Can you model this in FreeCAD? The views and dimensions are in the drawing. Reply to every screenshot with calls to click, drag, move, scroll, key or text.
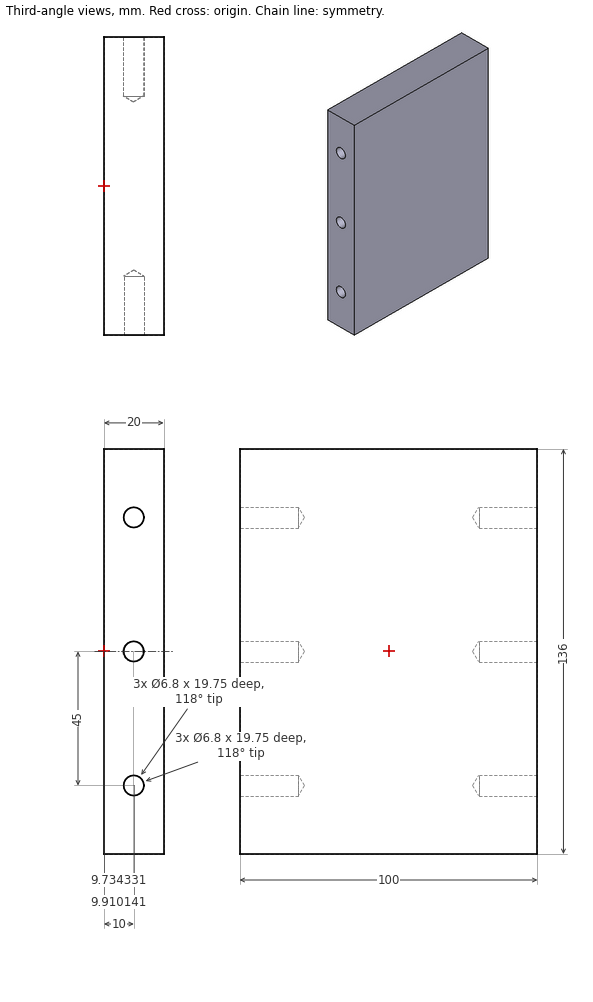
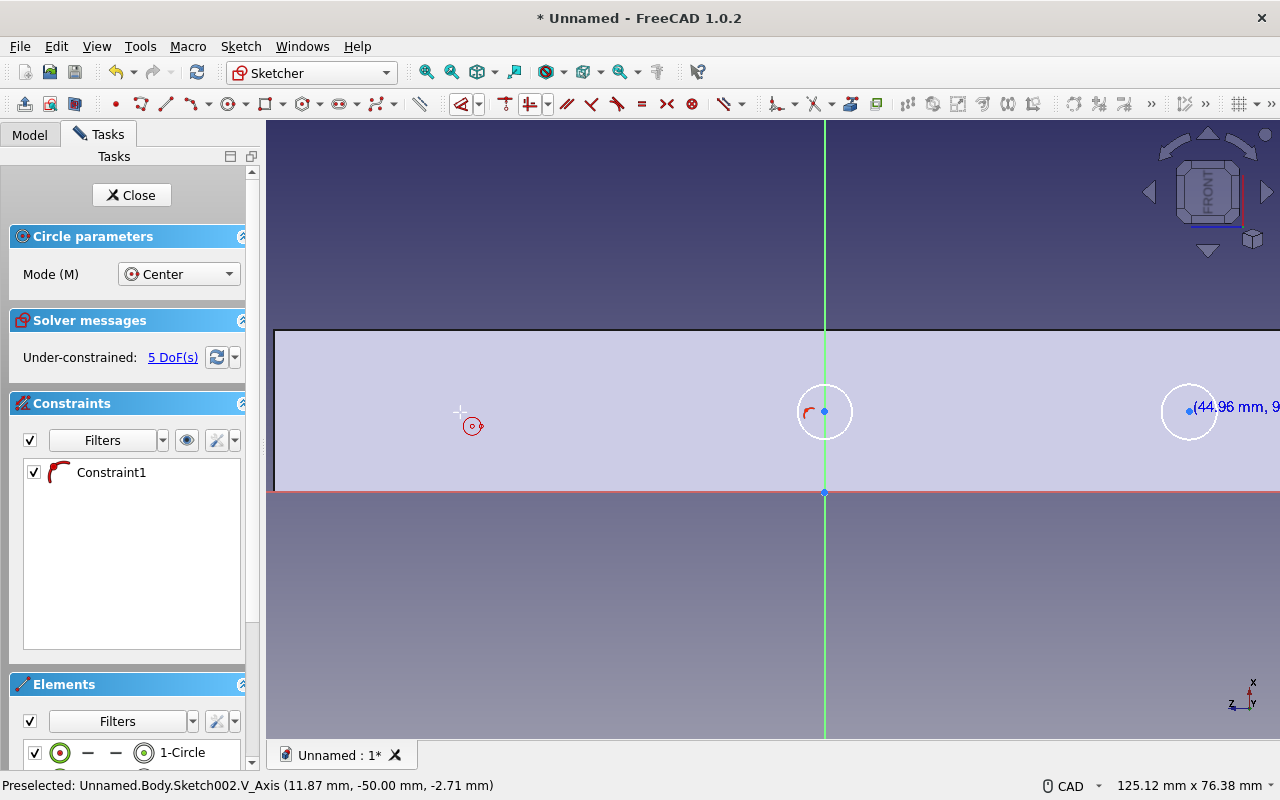
click(460, 411)
click(480, 392)
key(Escape)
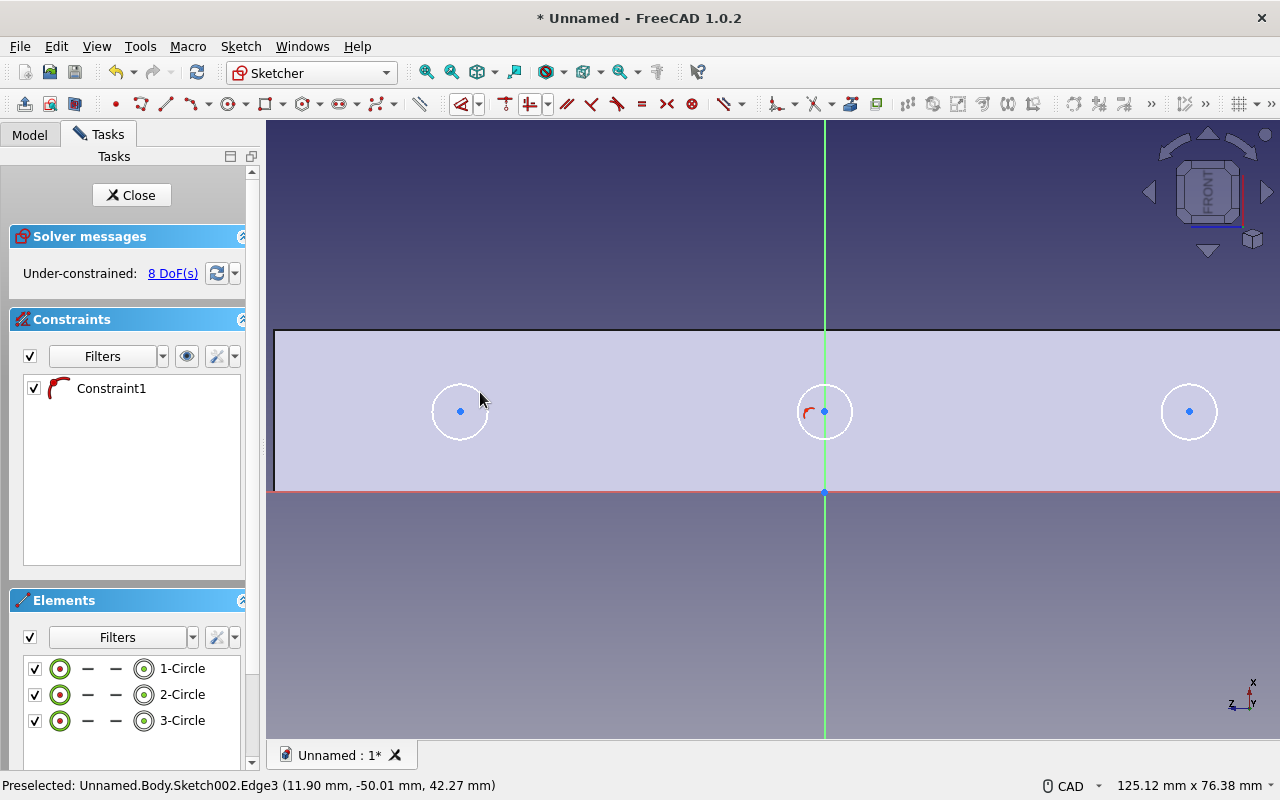
scroll(460, 412, down, 2)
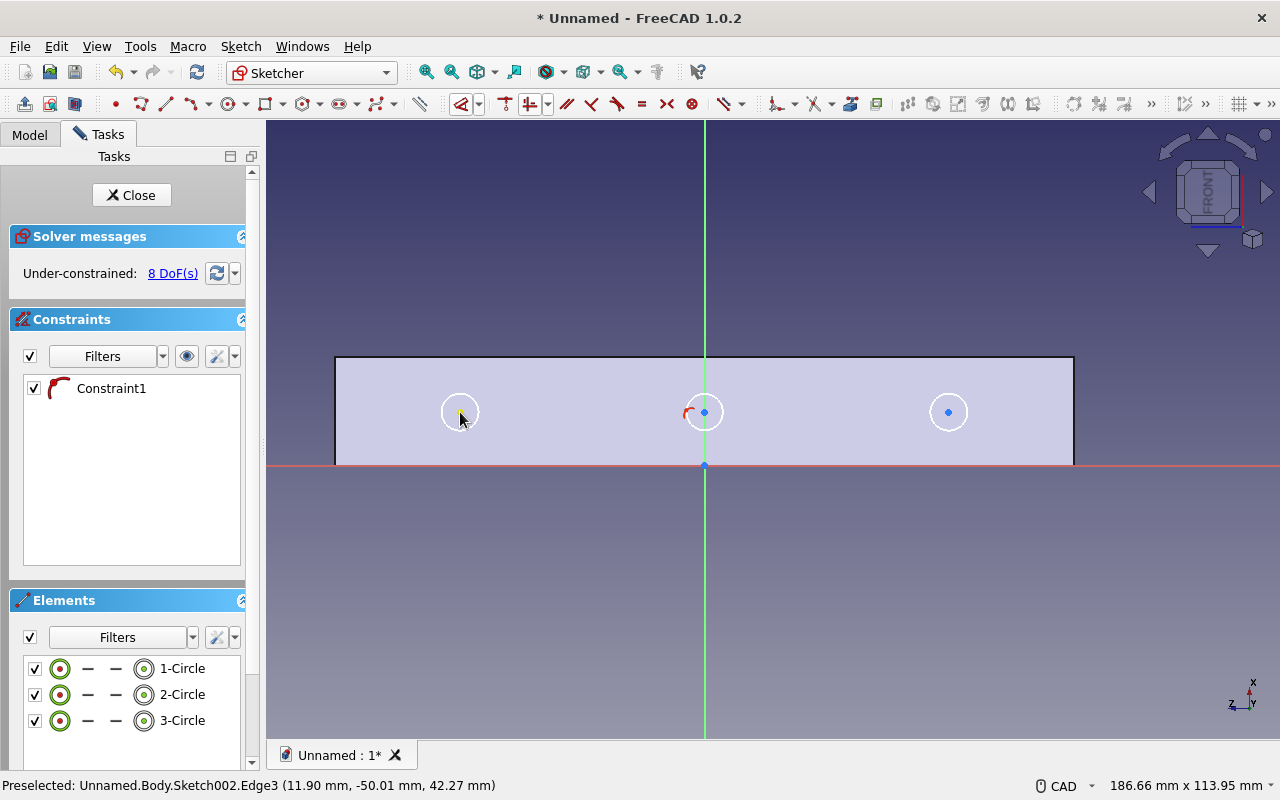
click(962, 399)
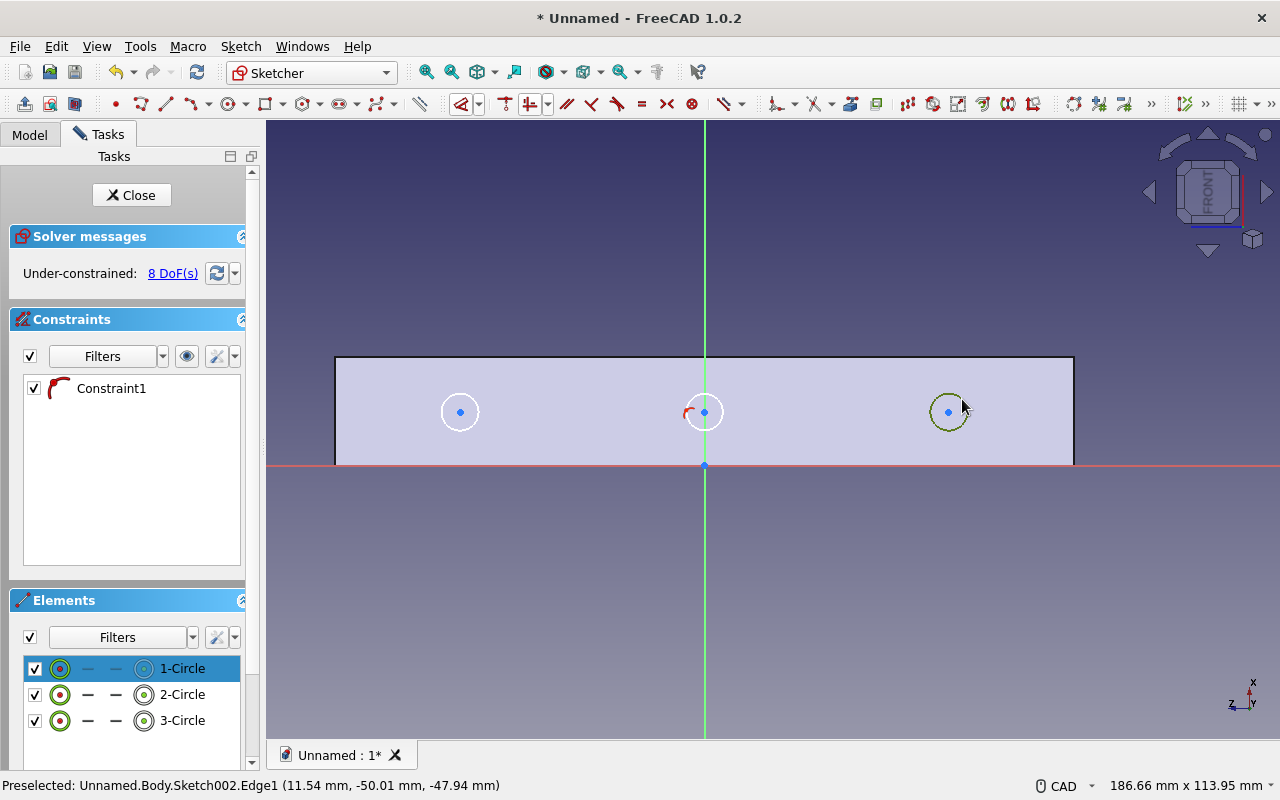
click(717, 399)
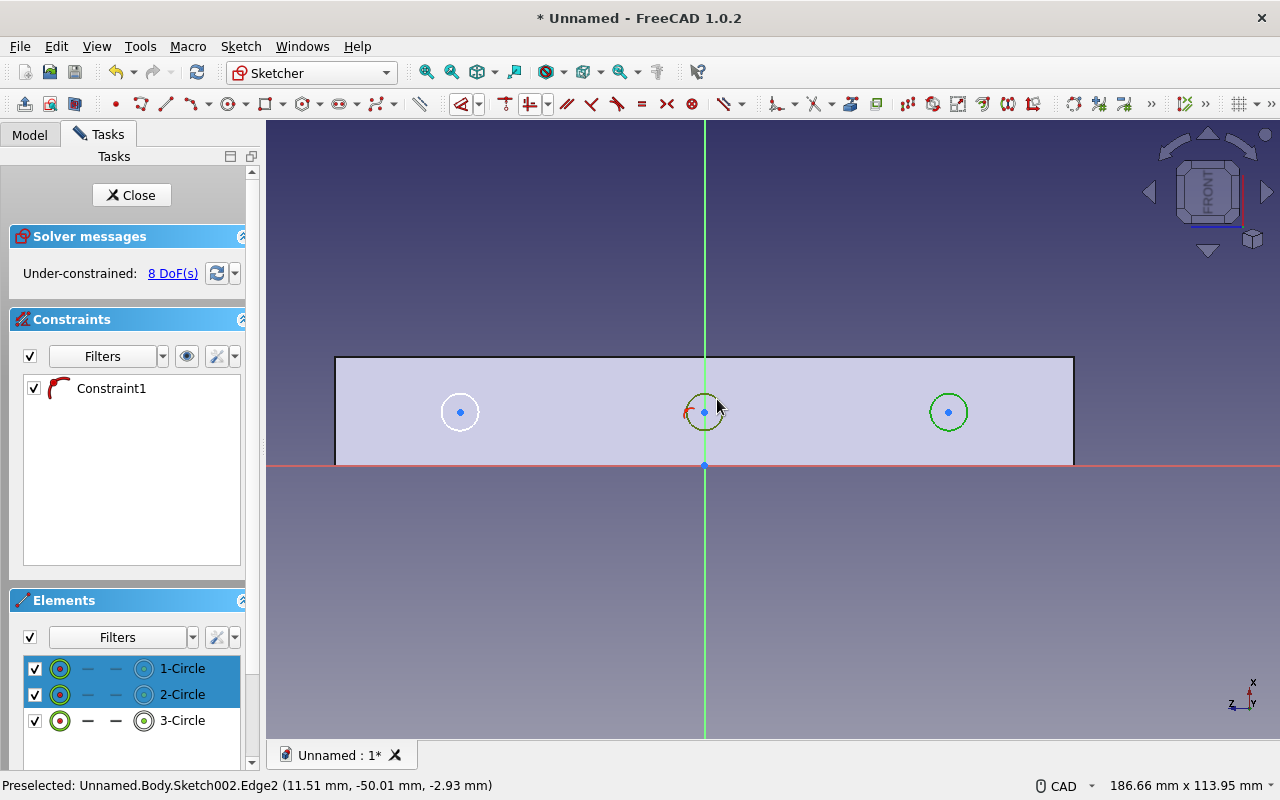
click(473, 399)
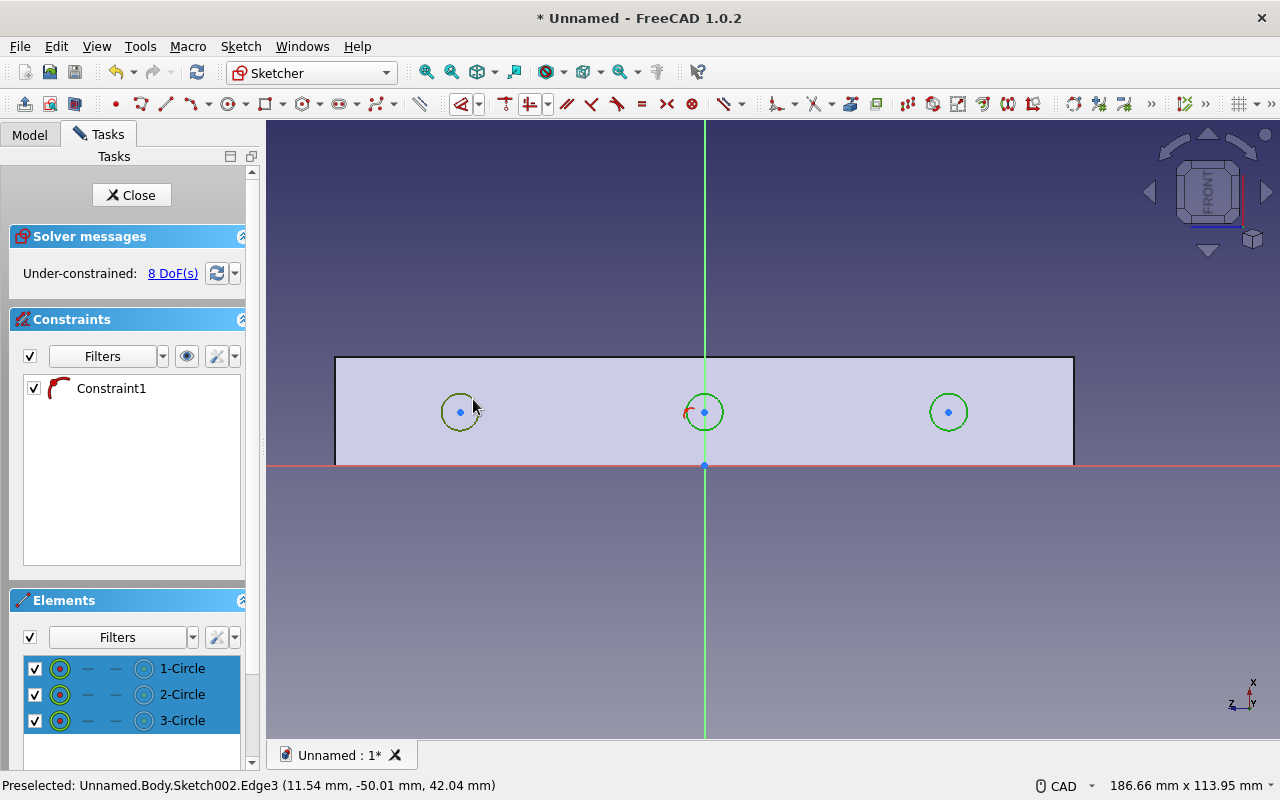
key(e)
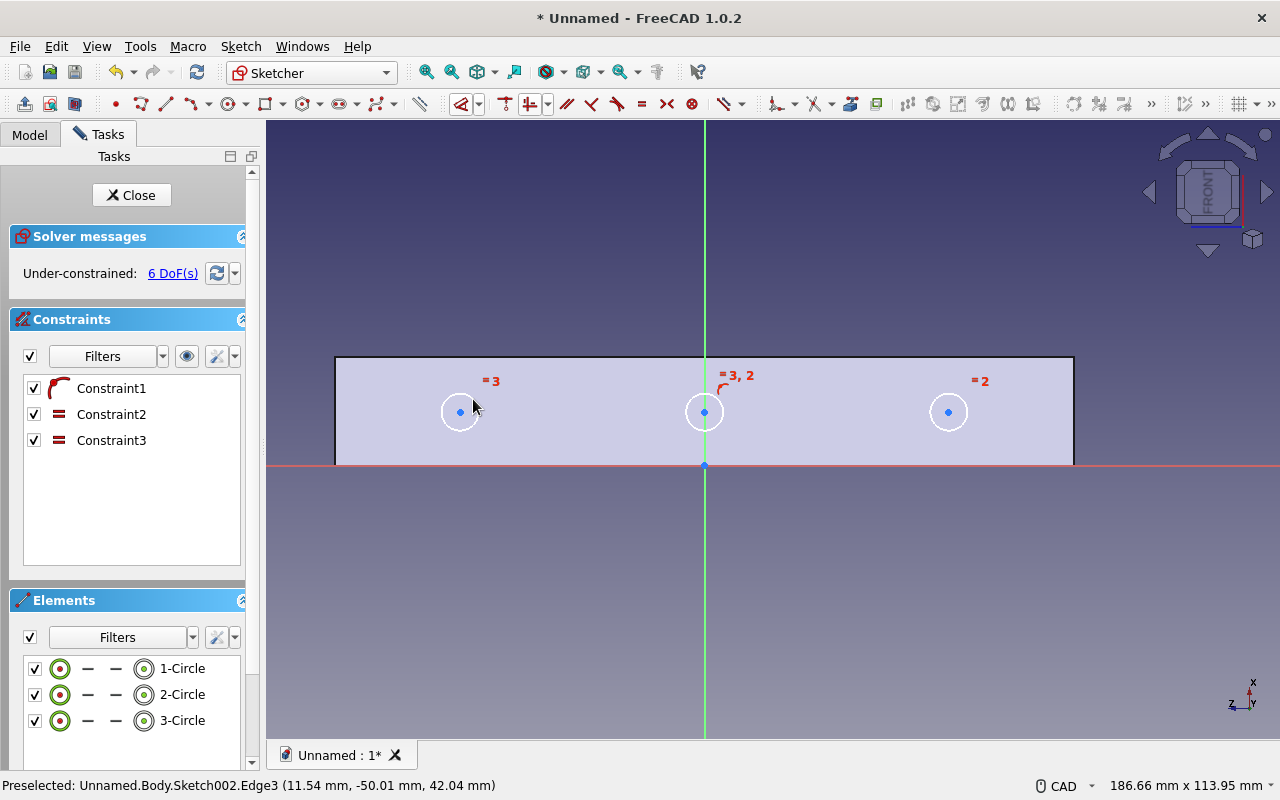
click(949, 412)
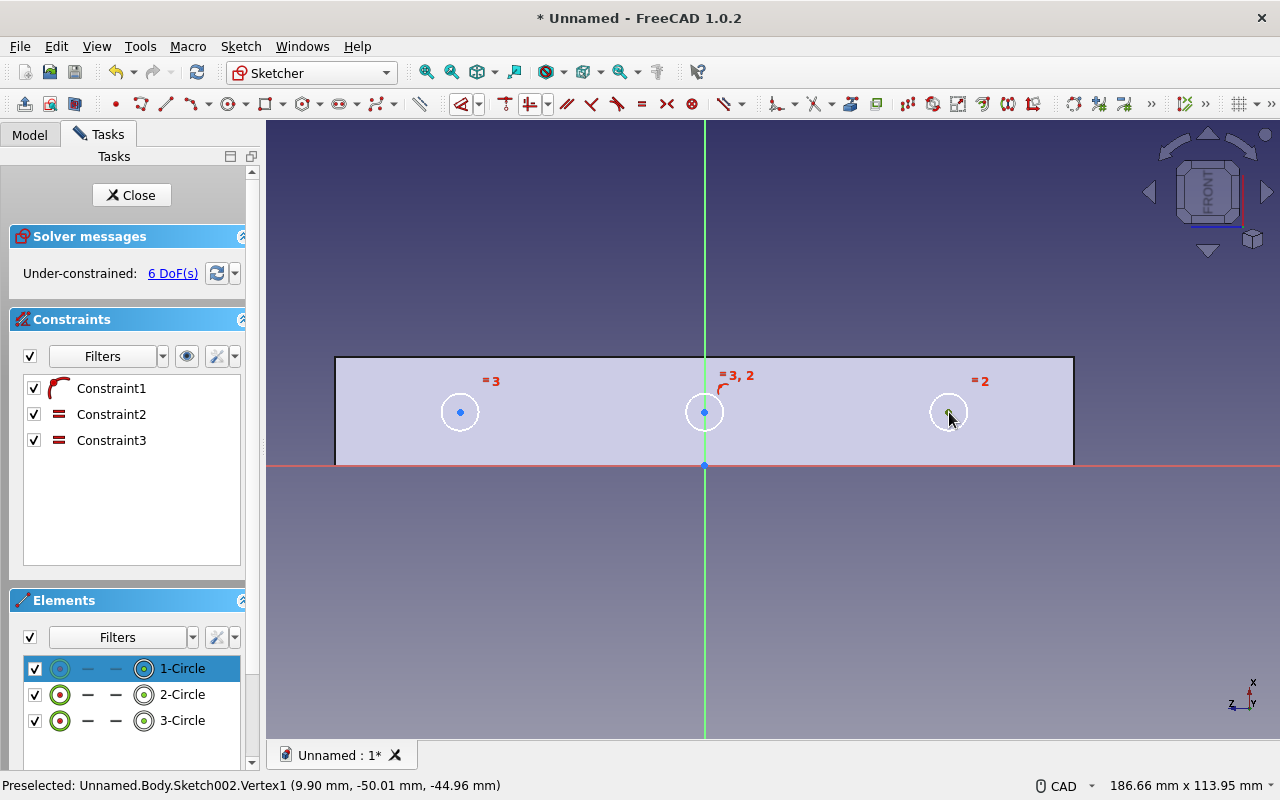
click(460, 412)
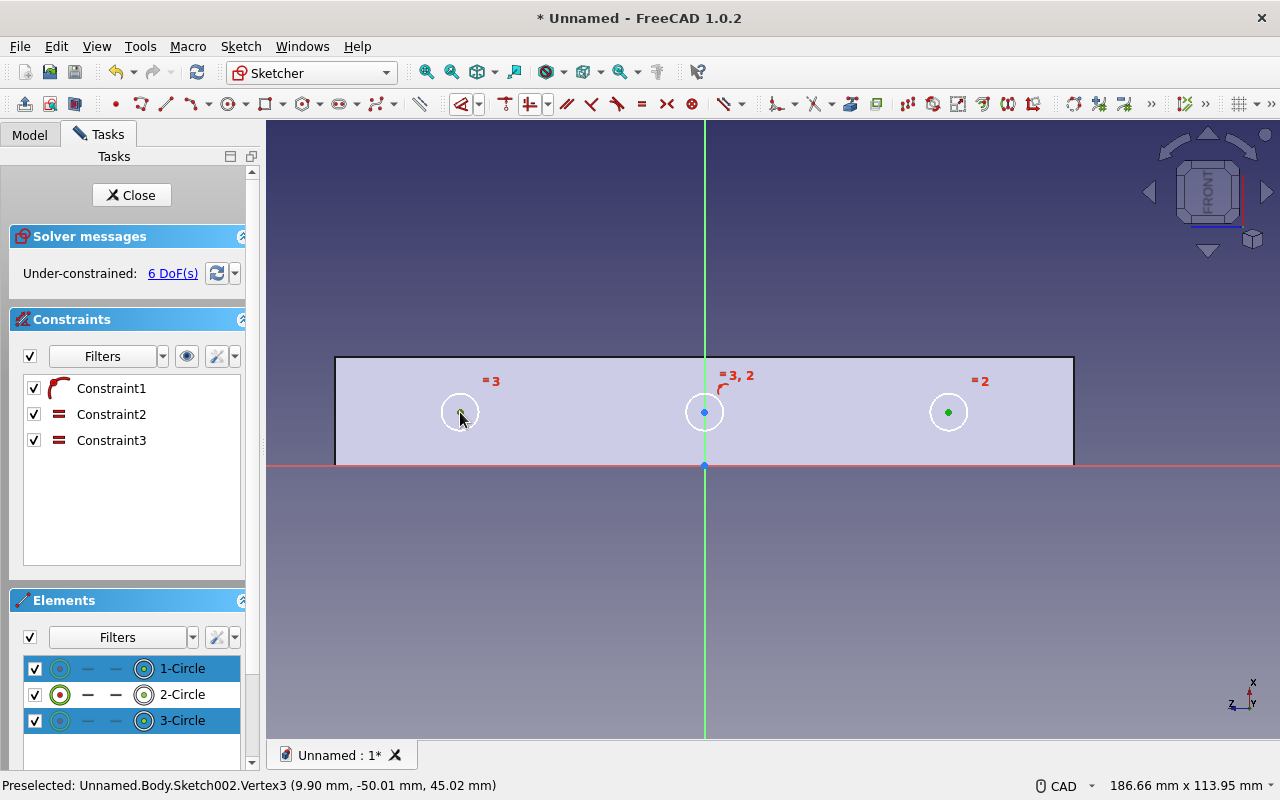
click(705, 671)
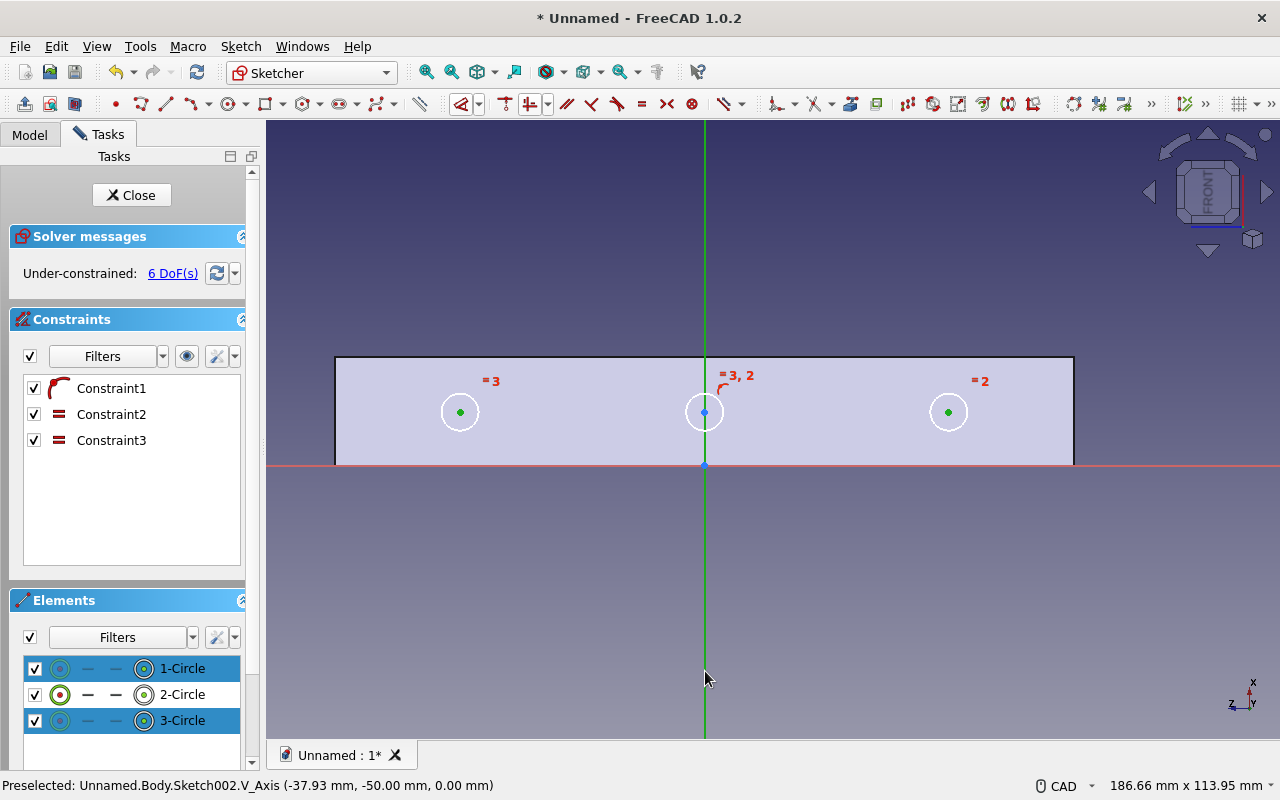
key(s)